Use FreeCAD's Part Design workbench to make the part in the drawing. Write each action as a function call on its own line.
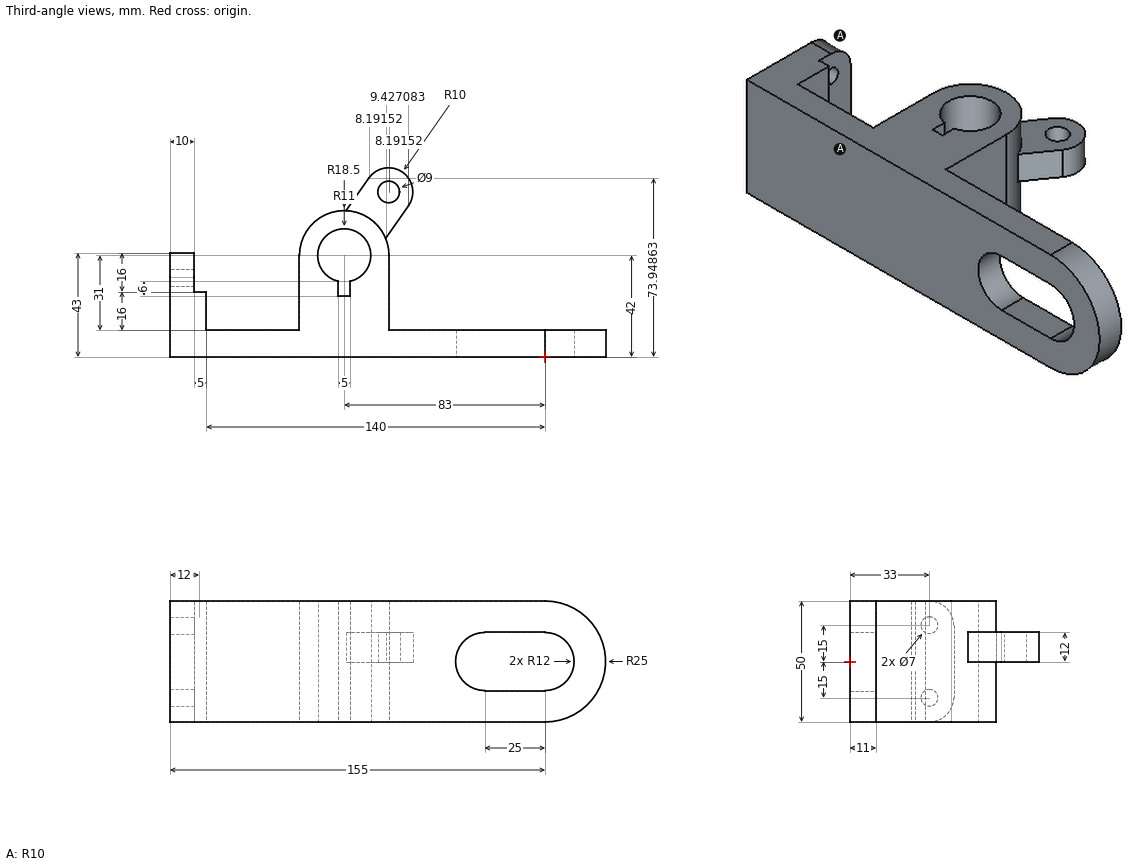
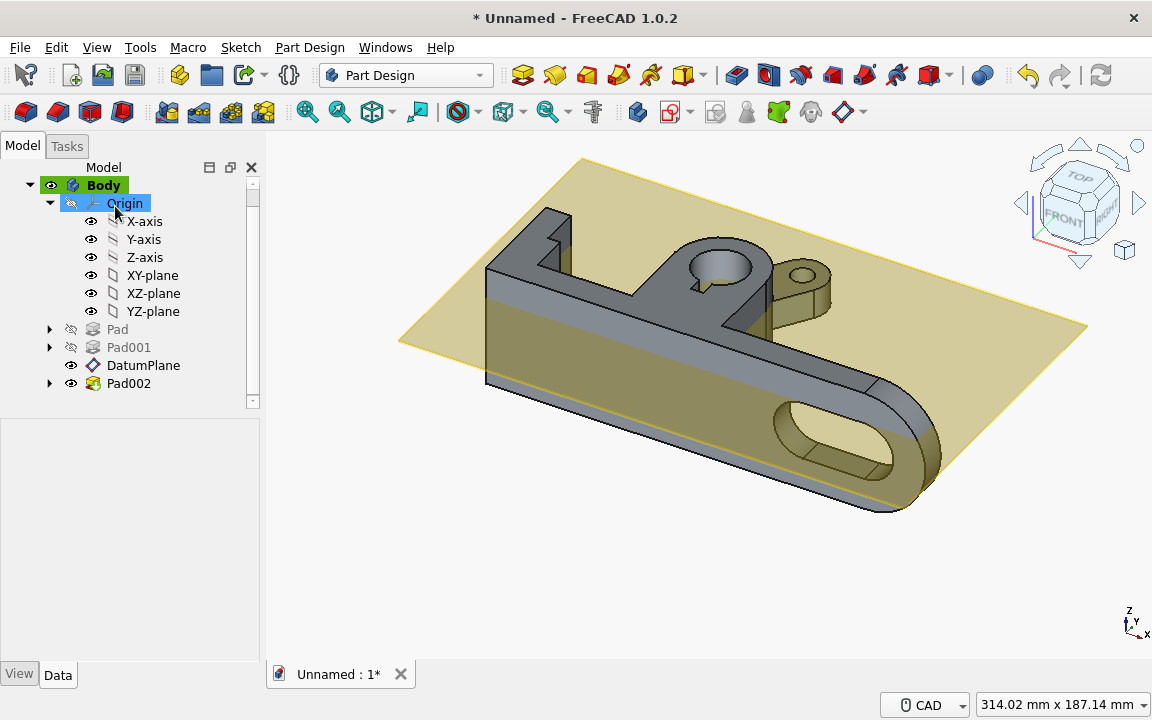
click(116, 365)
key(space)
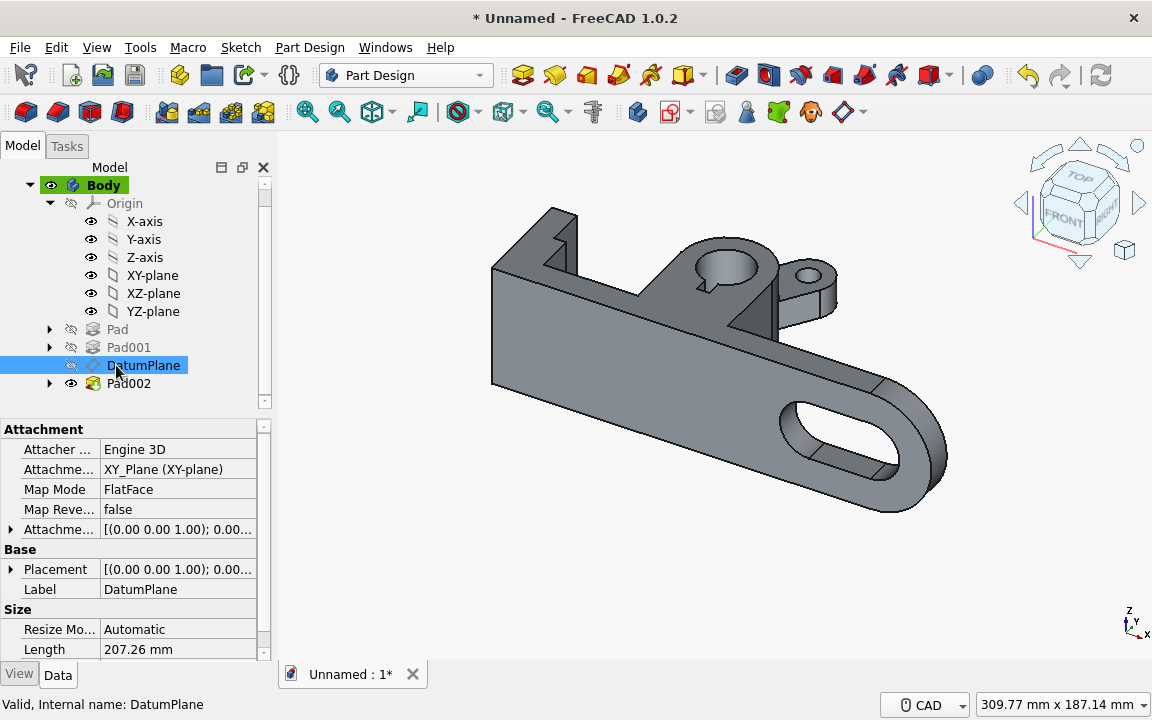
key(0)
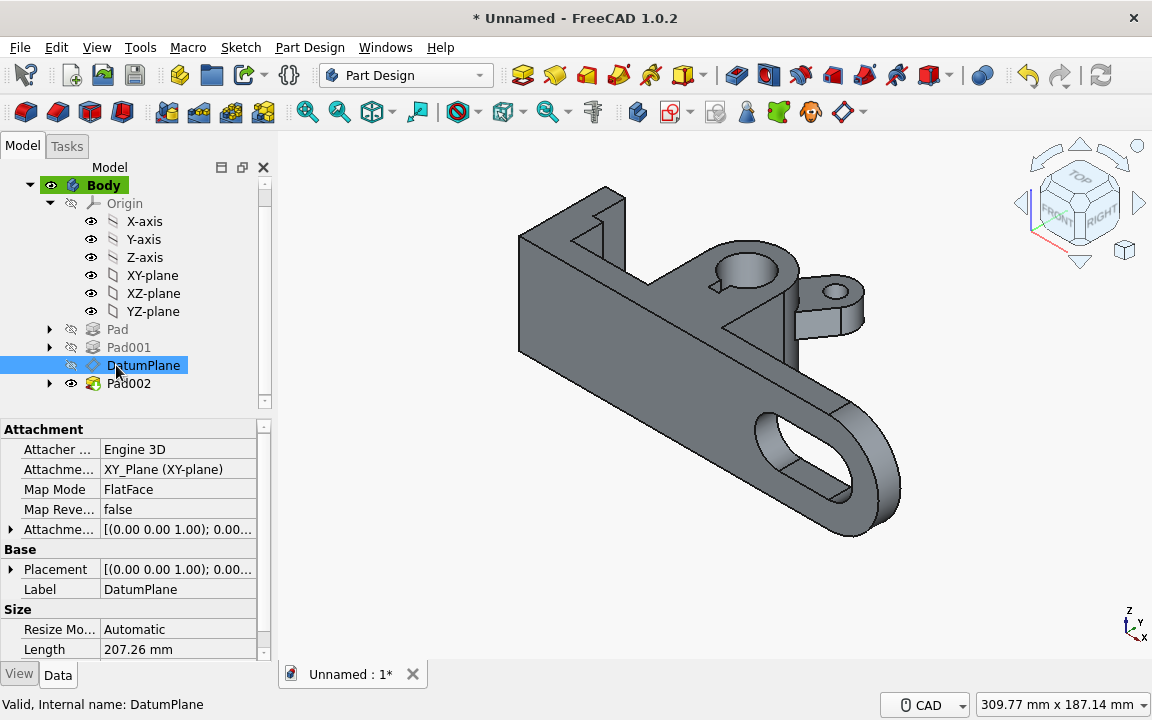
key(2)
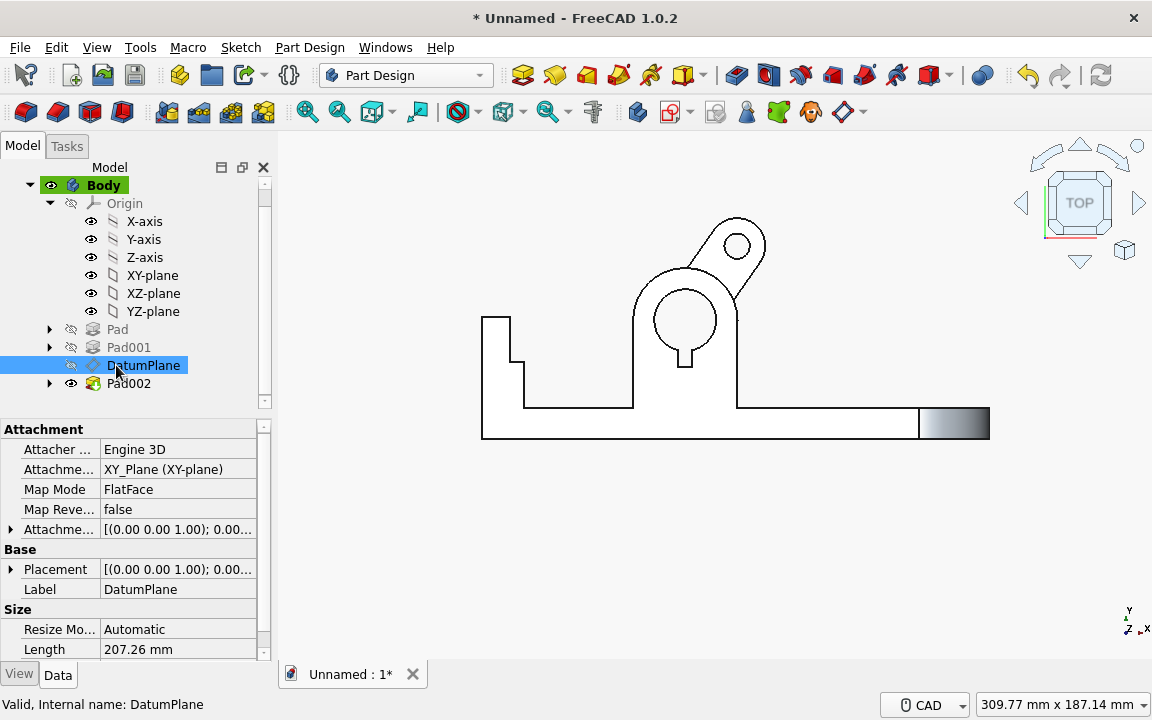
click(496, 316)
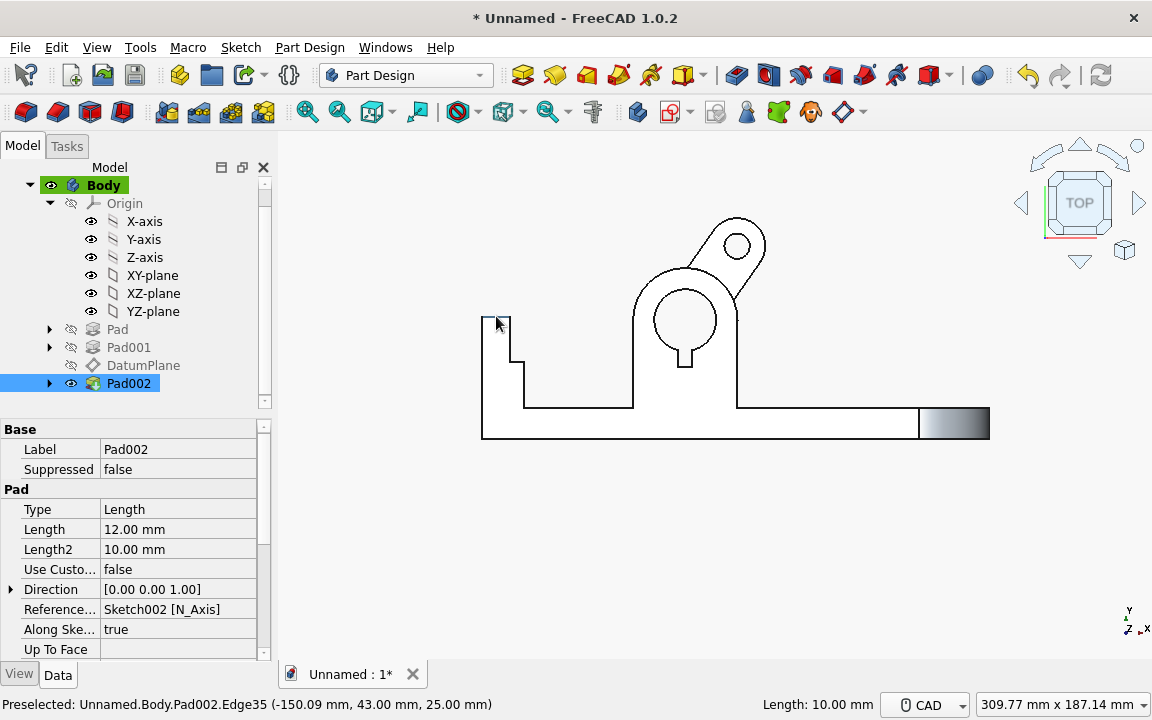
key(1)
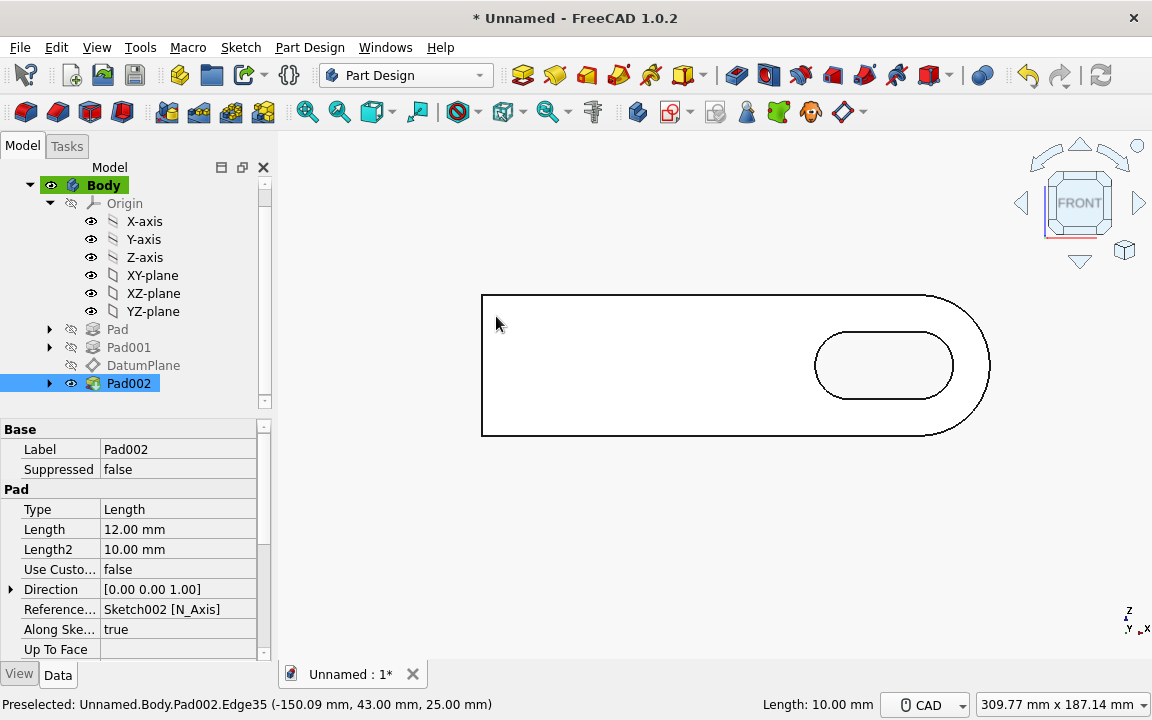
key(3)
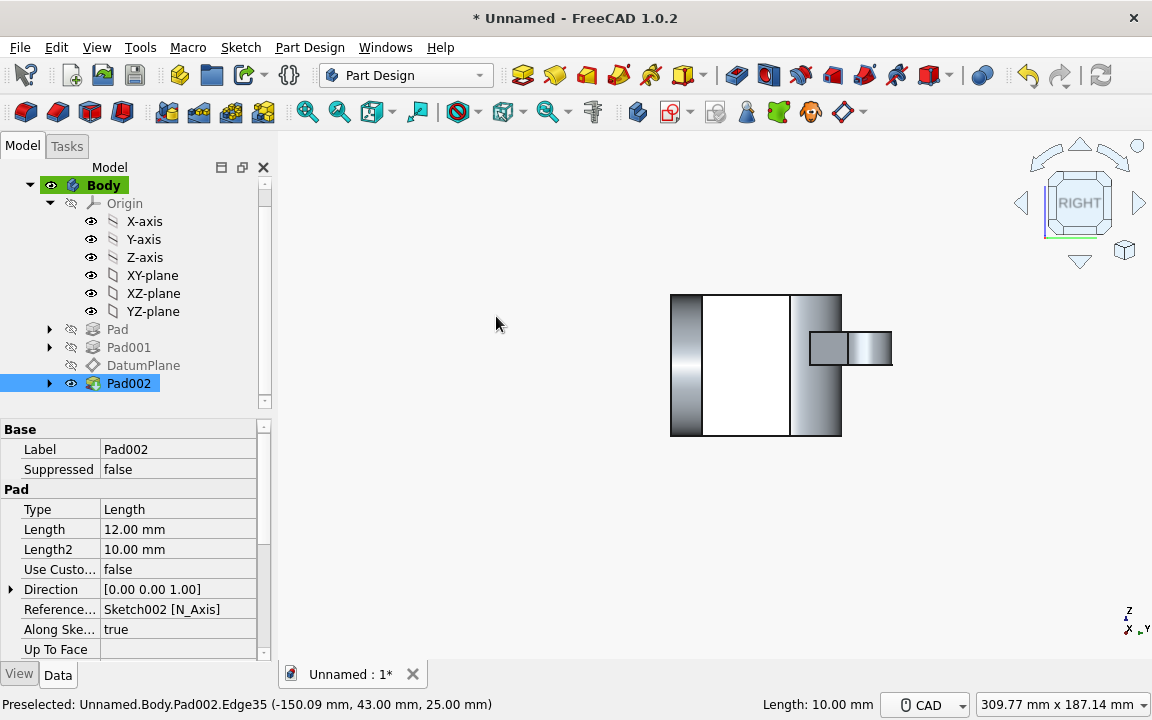
click(308, 112)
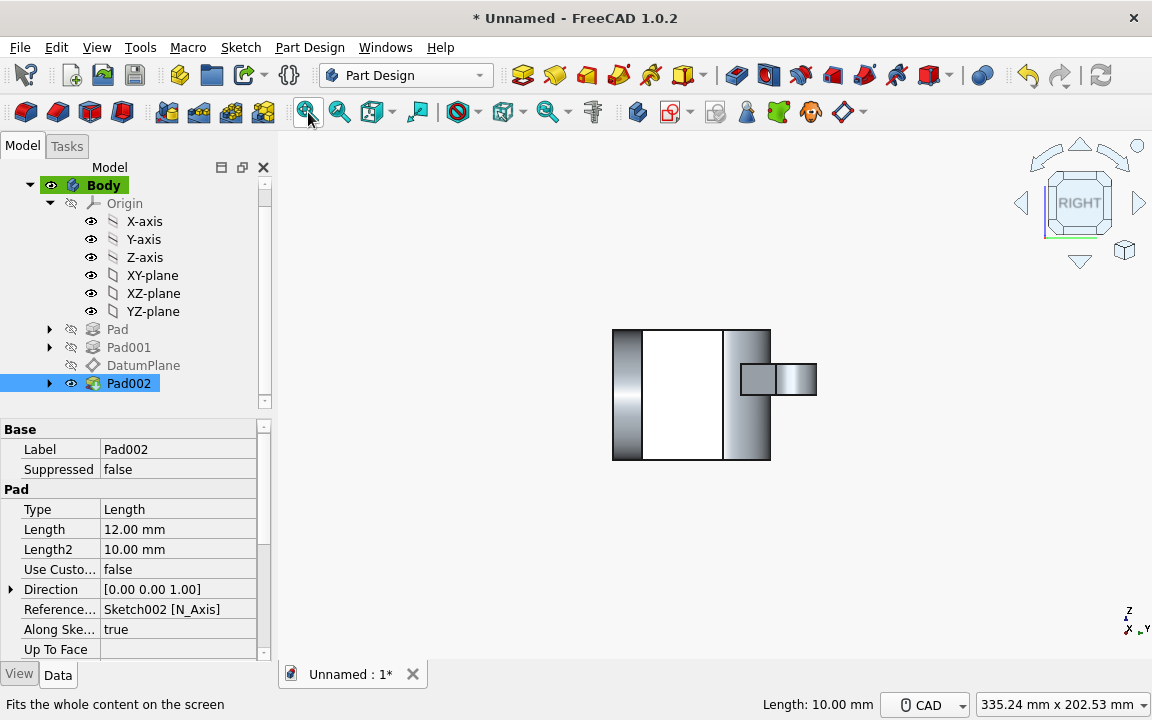
key(5)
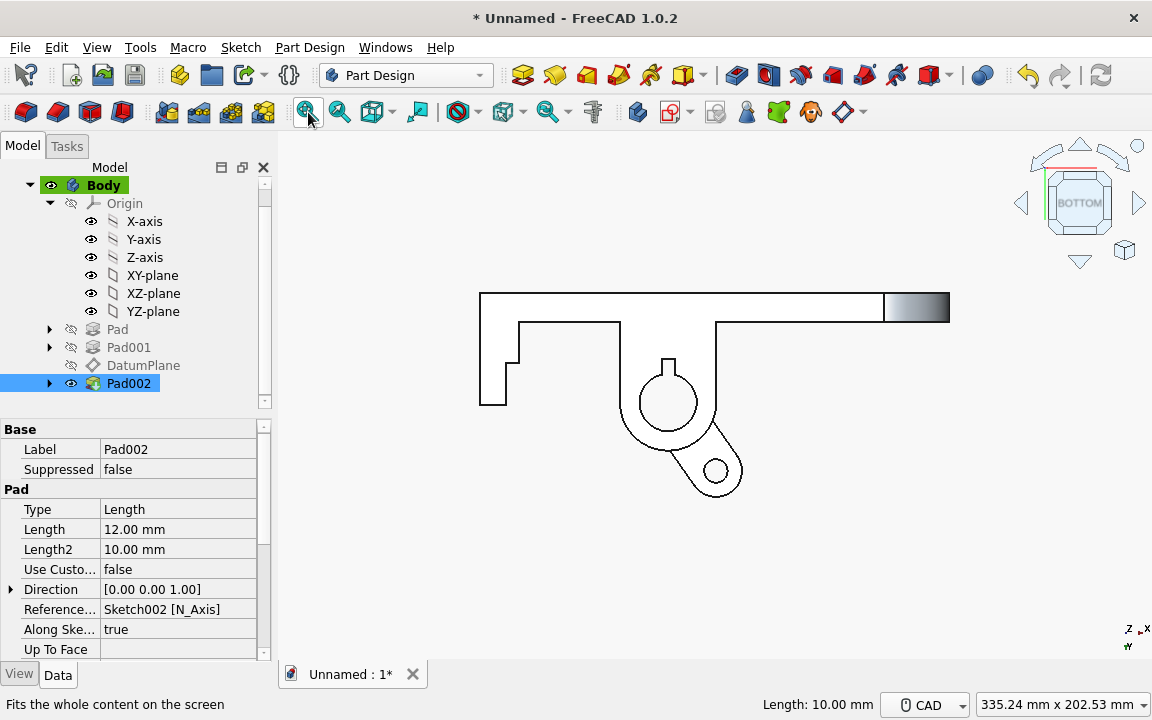
key(4)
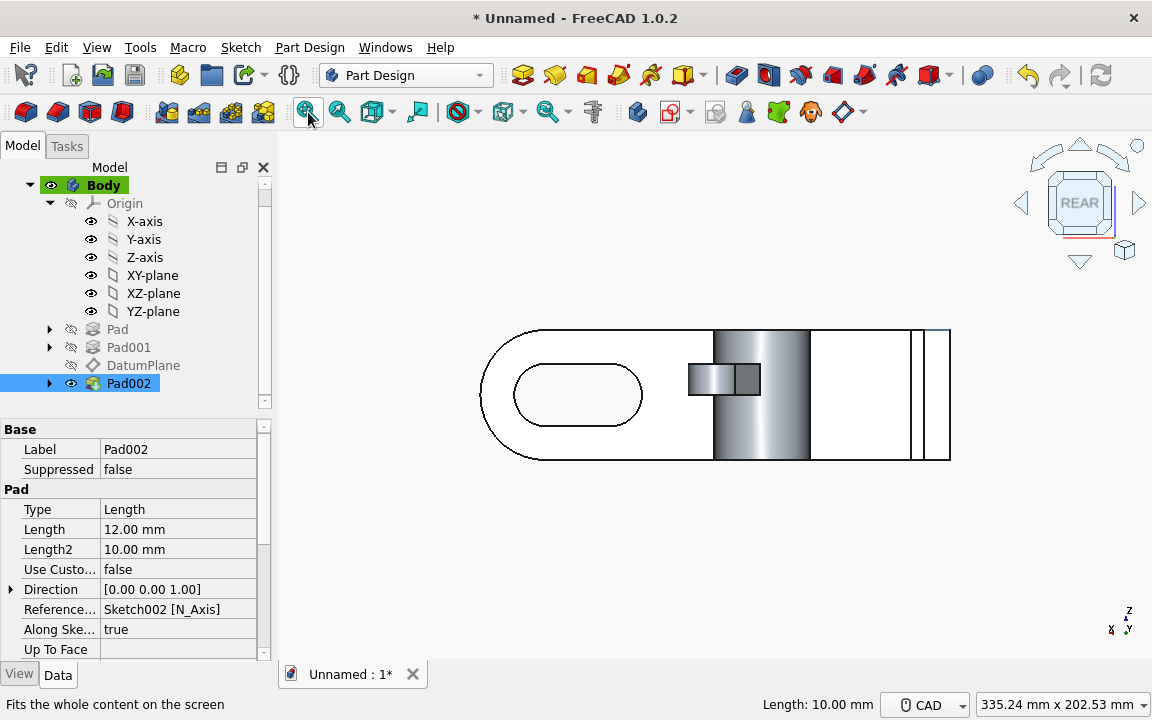
click(937, 459, ctrl)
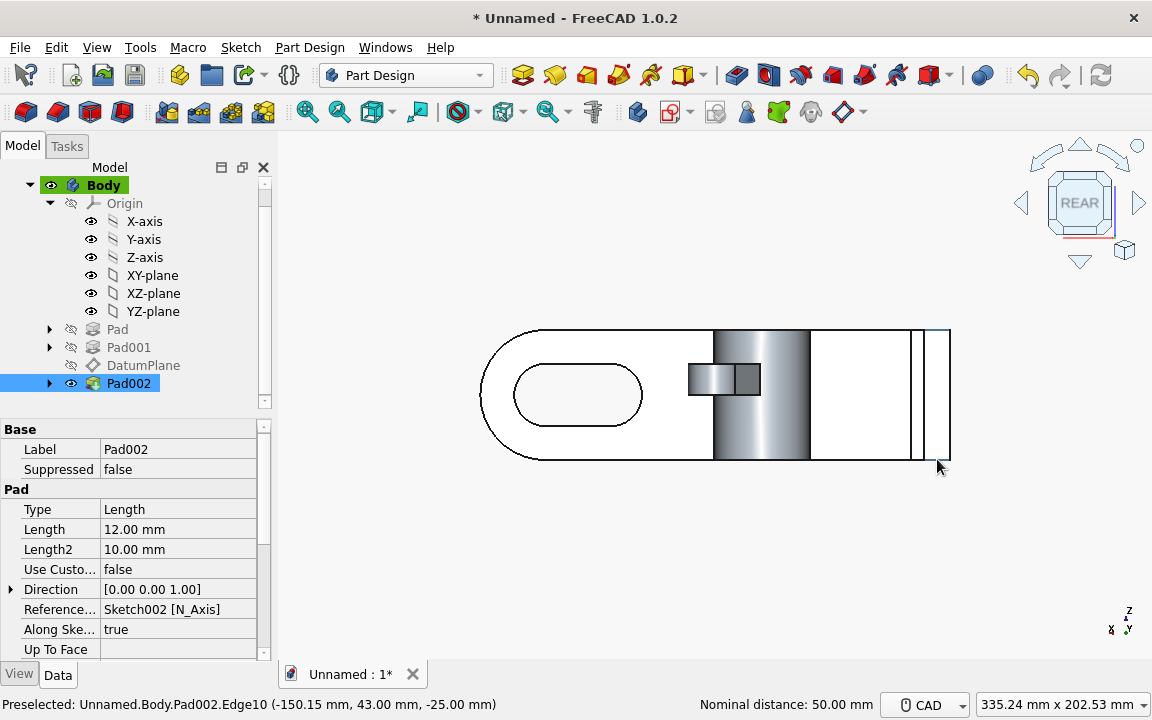
click(26, 112)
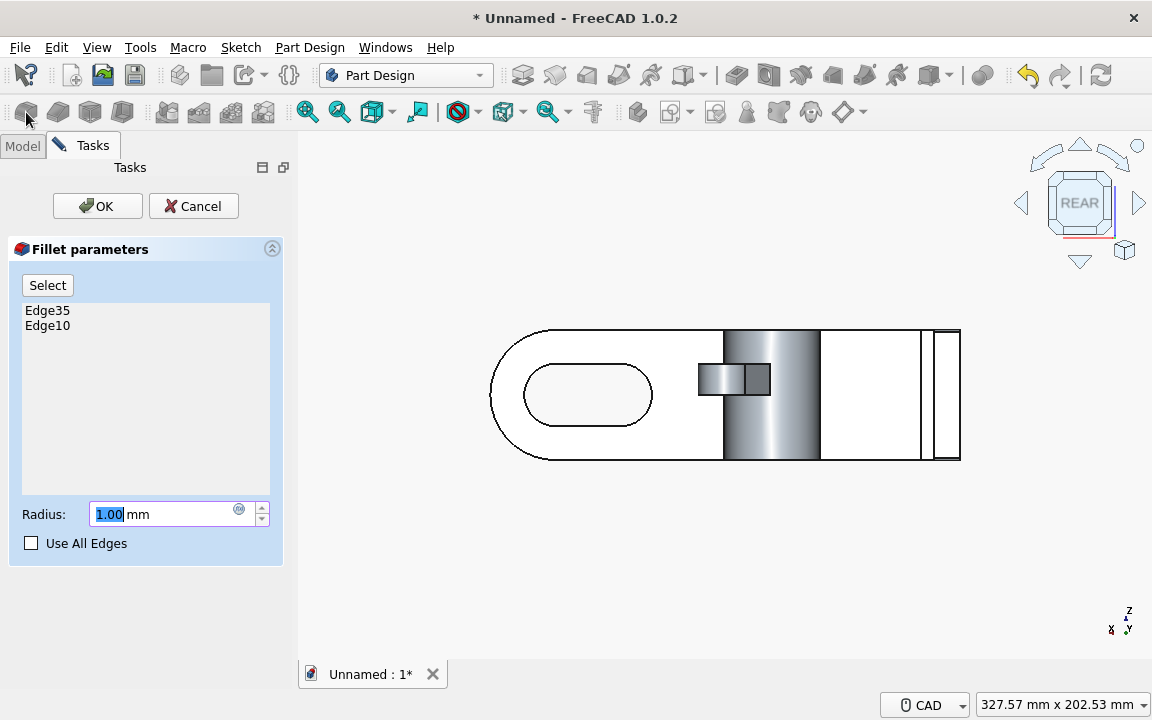
text(10)
key(Tab)